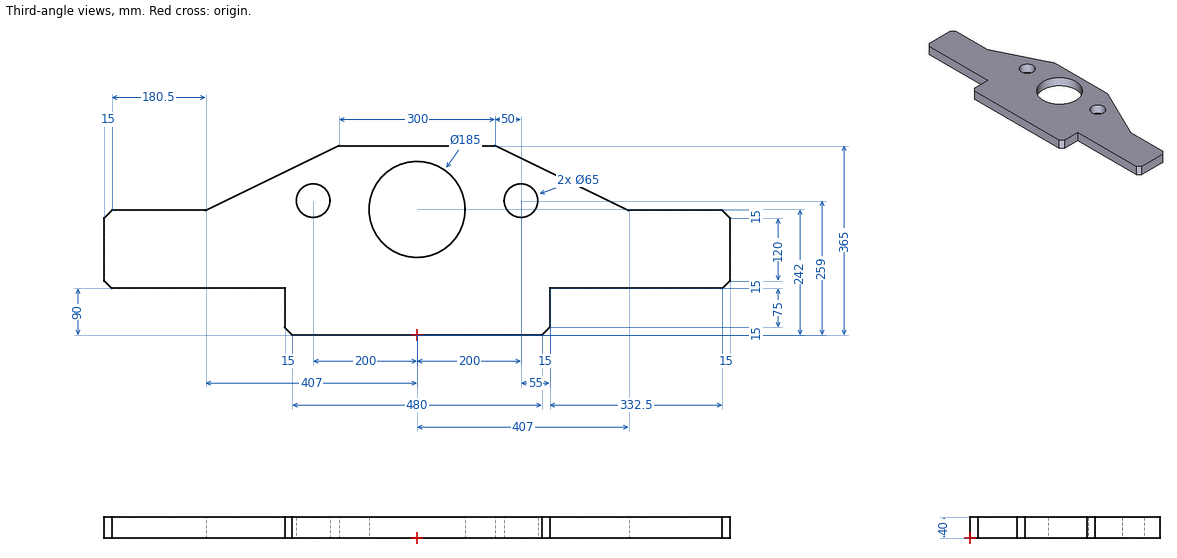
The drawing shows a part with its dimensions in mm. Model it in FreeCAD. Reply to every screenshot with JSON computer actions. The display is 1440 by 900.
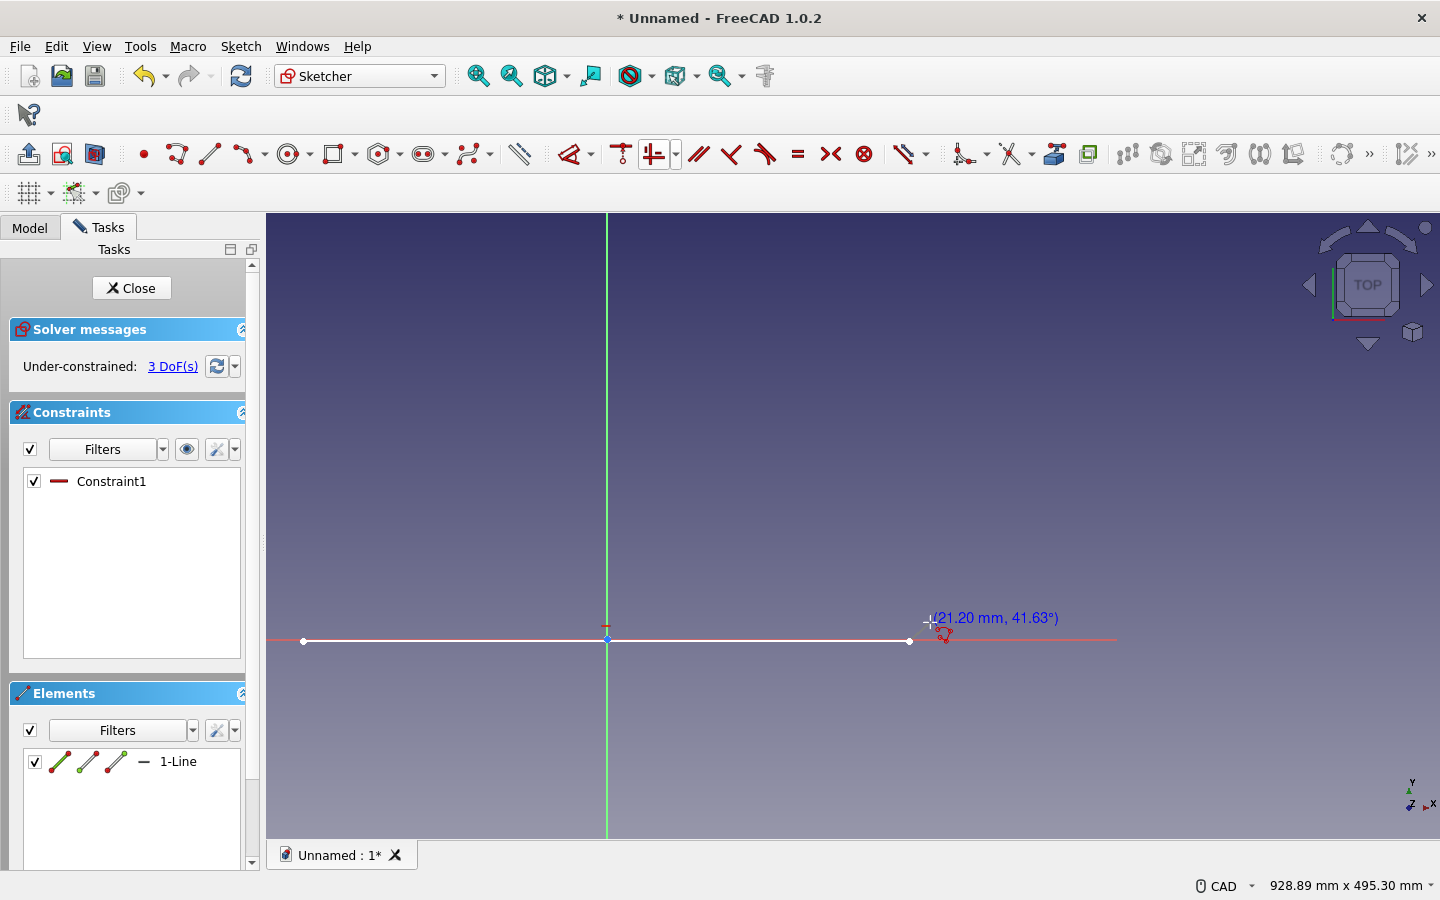
{"action": "left_click", "coordinate": [929, 621]}
{"action": "left_click", "coordinate": [929, 526]}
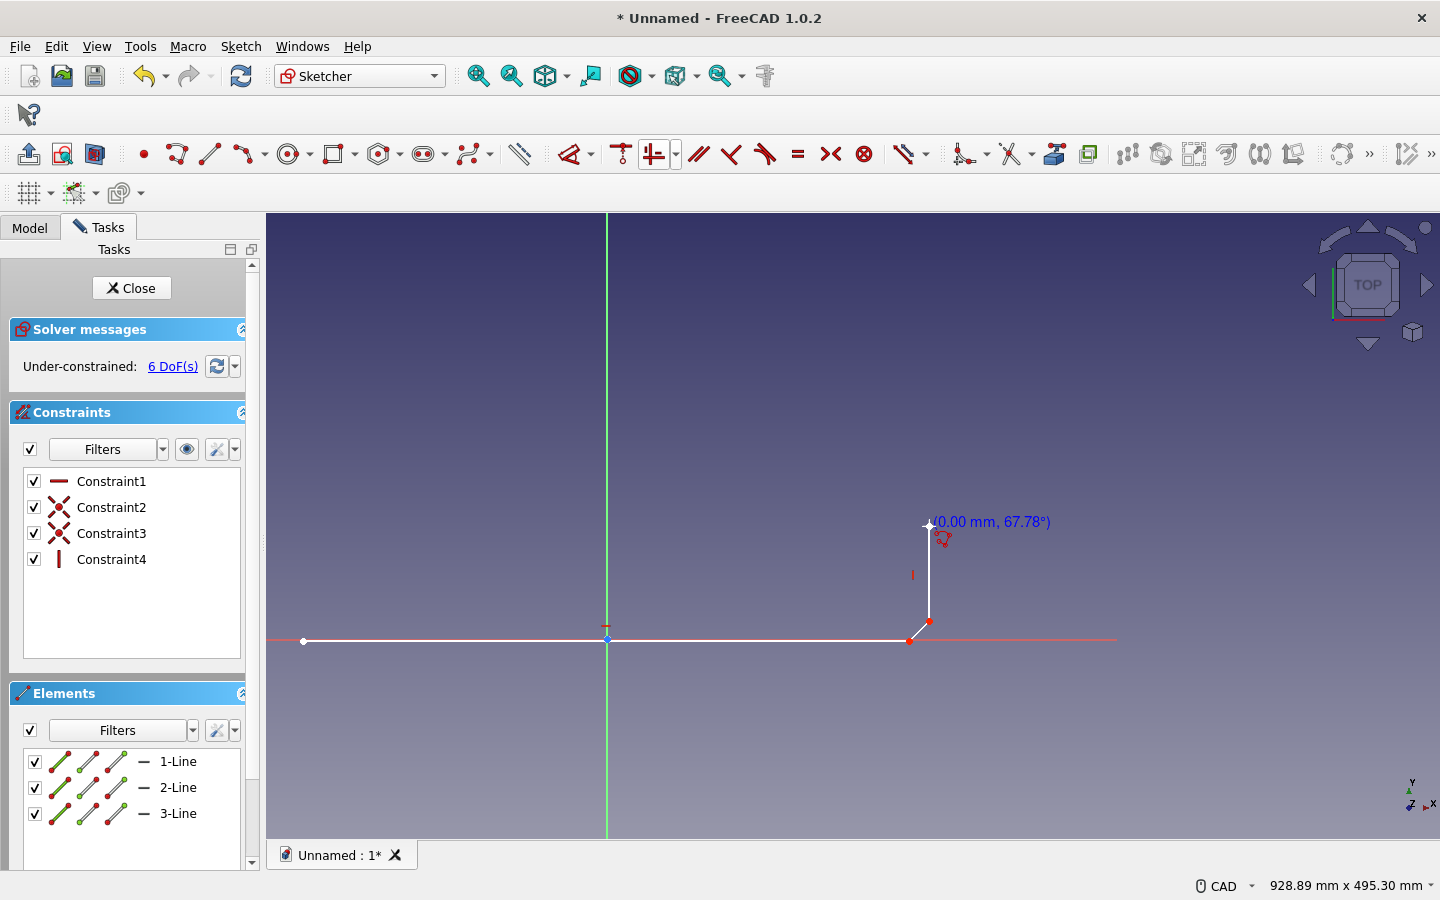
{"action": "scroll", "coordinate": [929, 621], "scroll_direction": "down", "scroll_amount": 4}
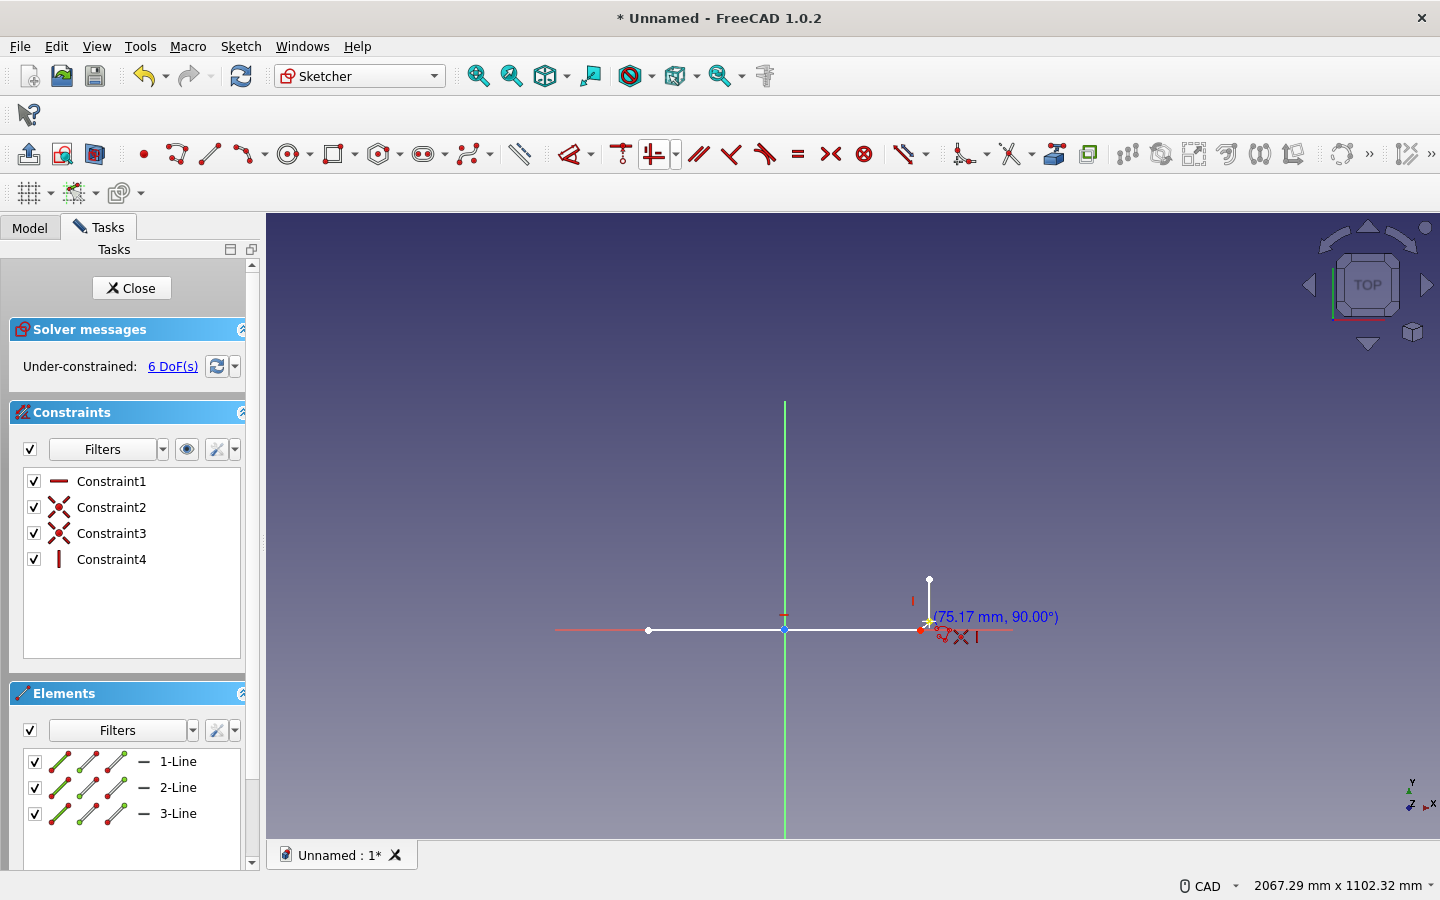
{"action": "left_click", "coordinate": [1118, 579]}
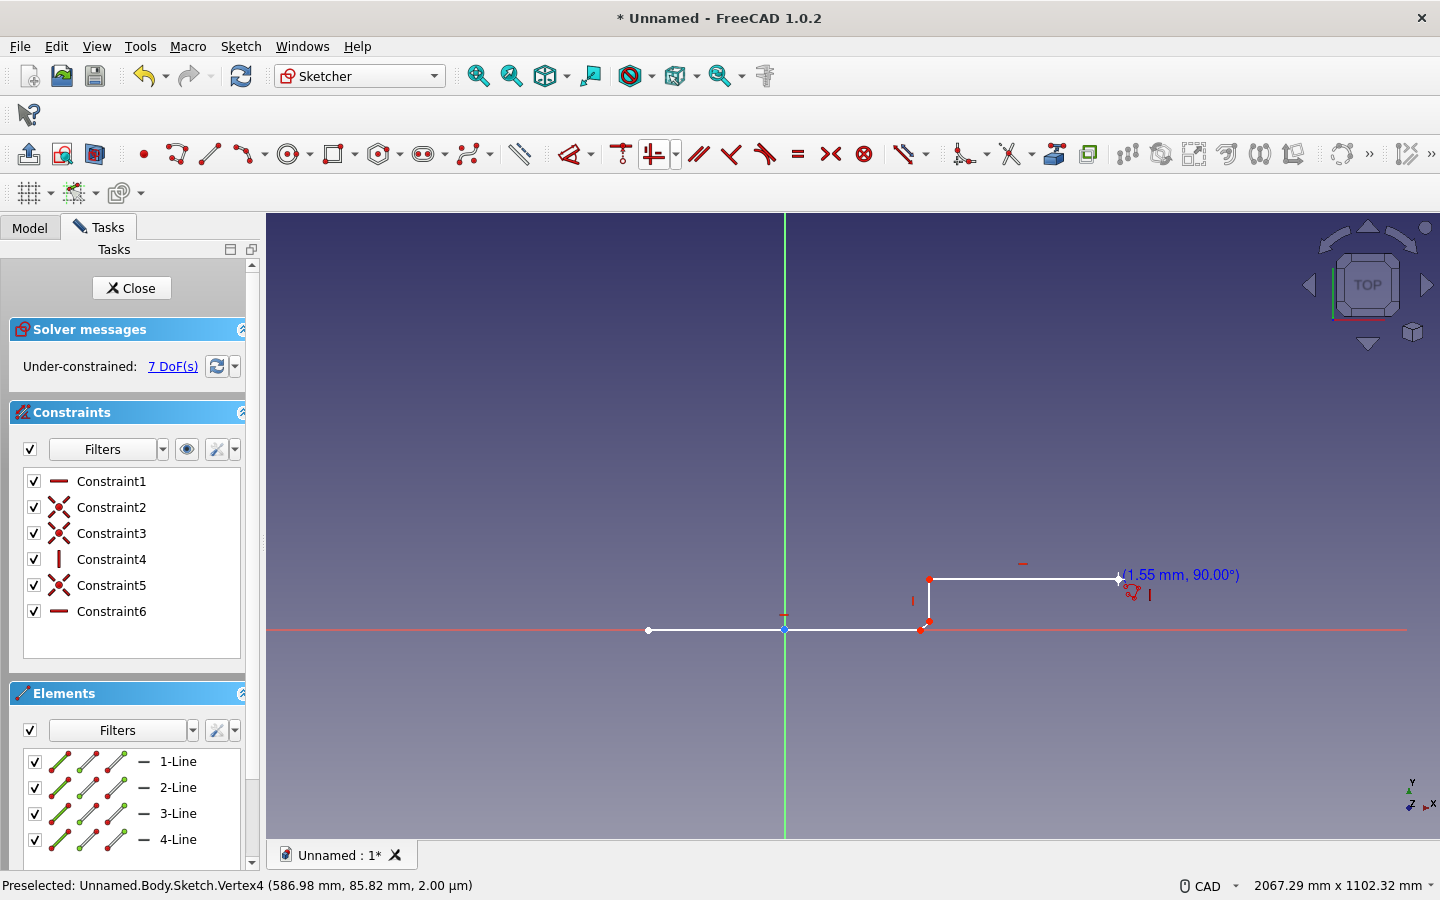
{"action": "scroll", "coordinate": [1127, 570], "scroll_direction": "up", "scroll_amount": 2}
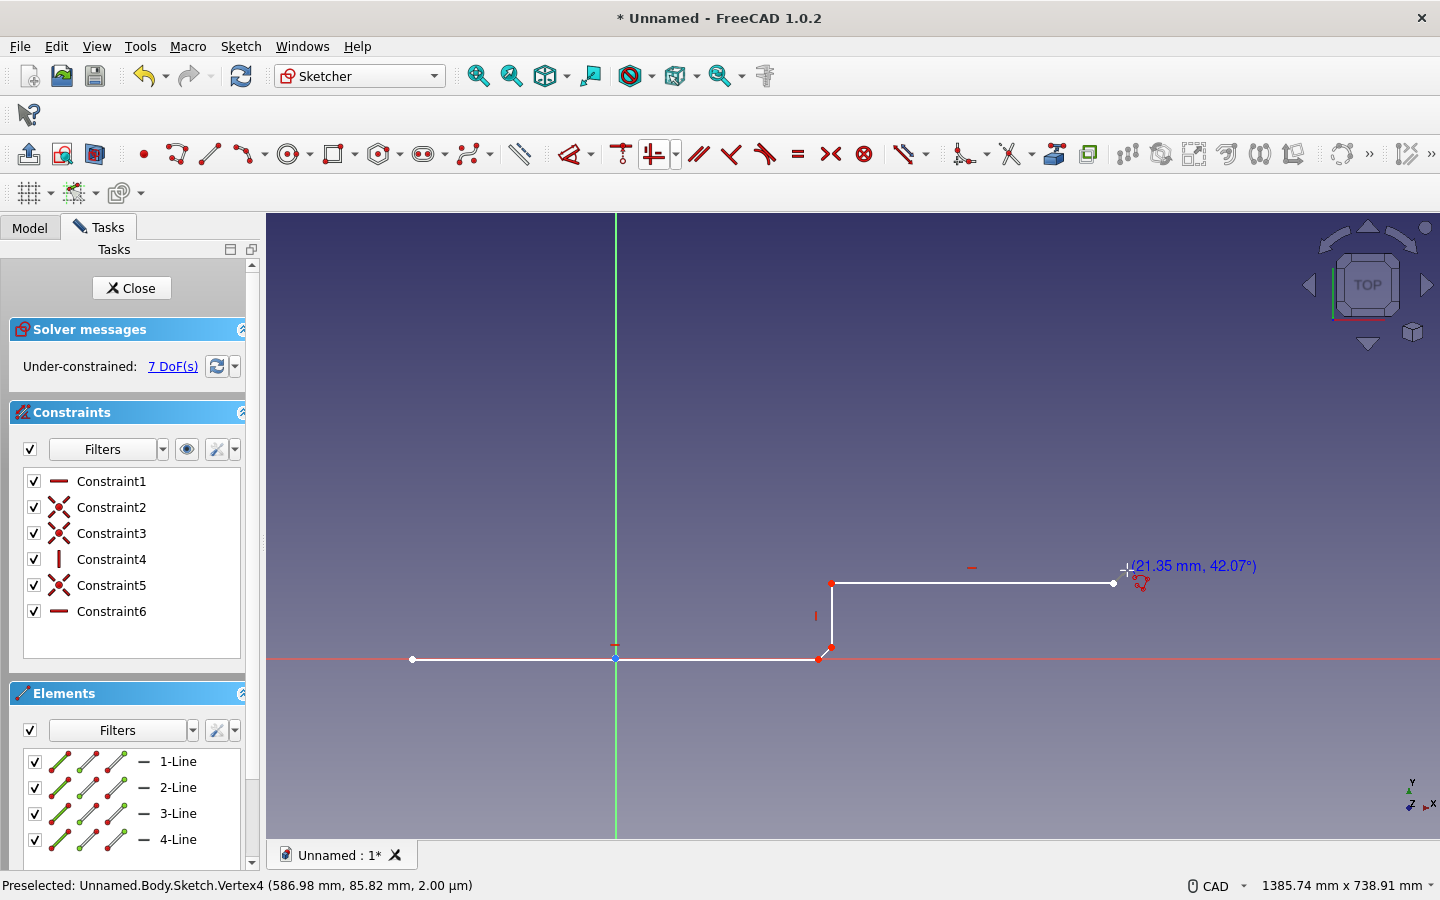
{"action": "left_click", "coordinate": [1126, 570]}
{"action": "left_click", "coordinate": [1126, 468]}
{"action": "left_click", "coordinate": [1114, 455]}
{"action": "left_click", "coordinate": [961, 455]}
{"action": "left_click", "coordinate": [743, 350]}
{"action": "left_click", "coordinate": [489, 350]}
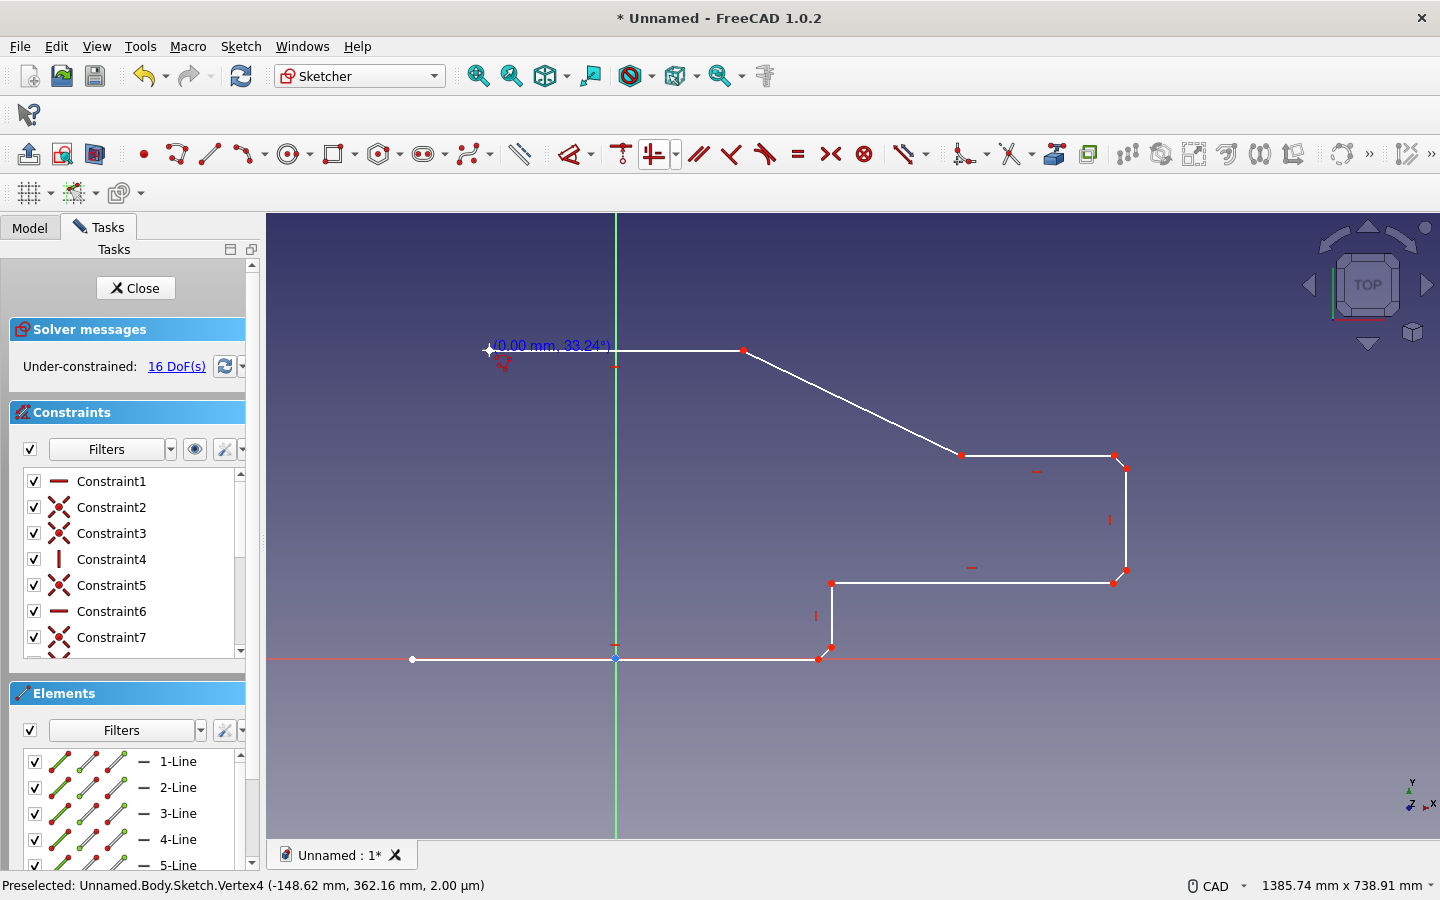
{"action": "scroll", "coordinate": [1127, 570], "scroll_direction": "down", "scroll_amount": 2}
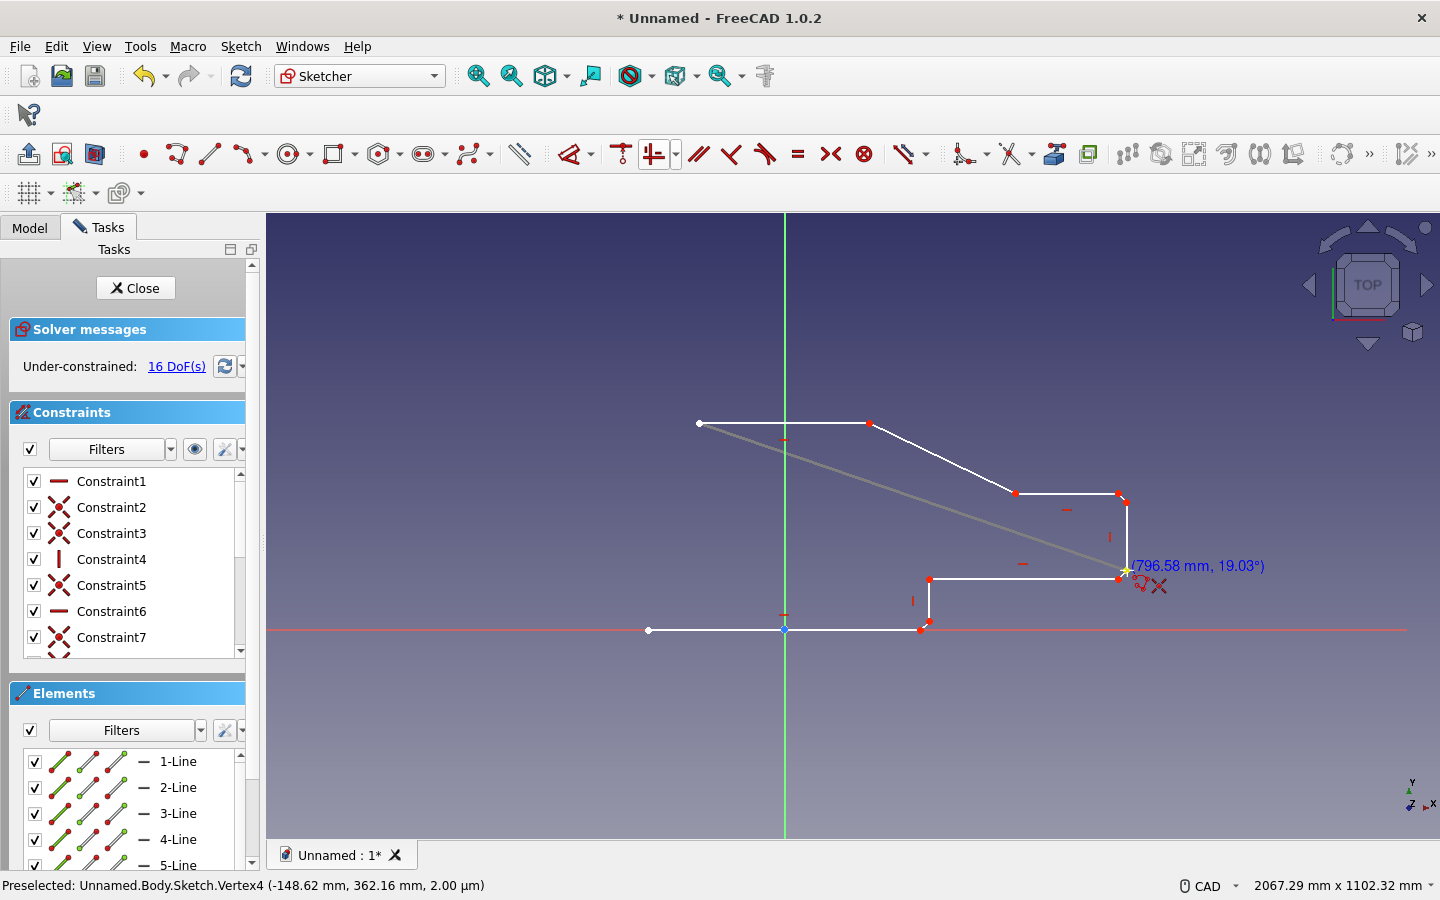
{"action": "left_click", "coordinate": [554, 493]}
{"action": "left_click", "coordinate": [451, 493]}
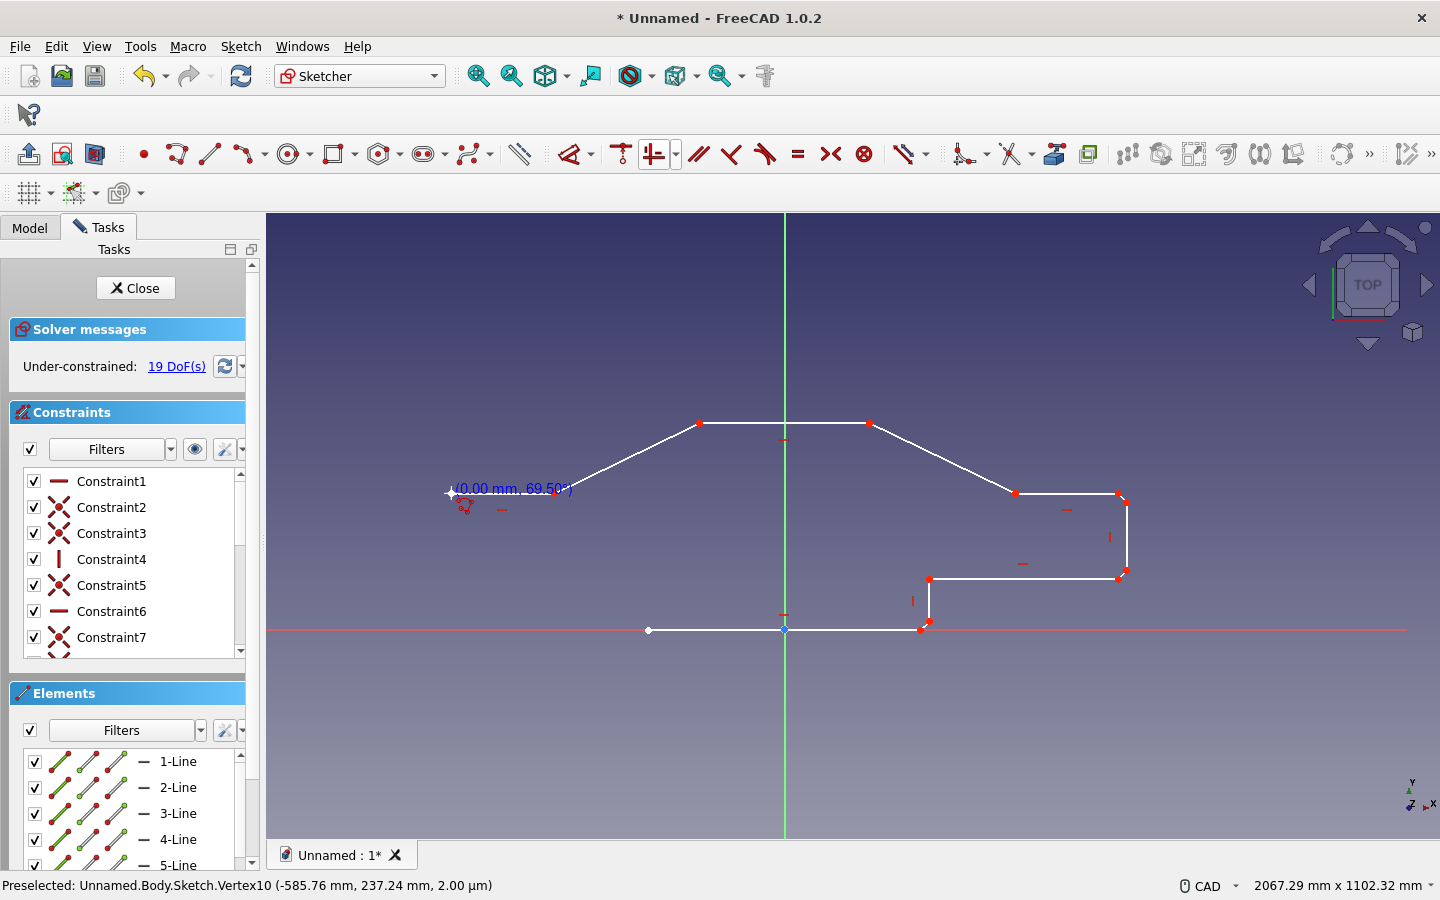
{"action": "scroll", "coordinate": [442, 502], "scroll_direction": "up", "scroll_amount": 2}